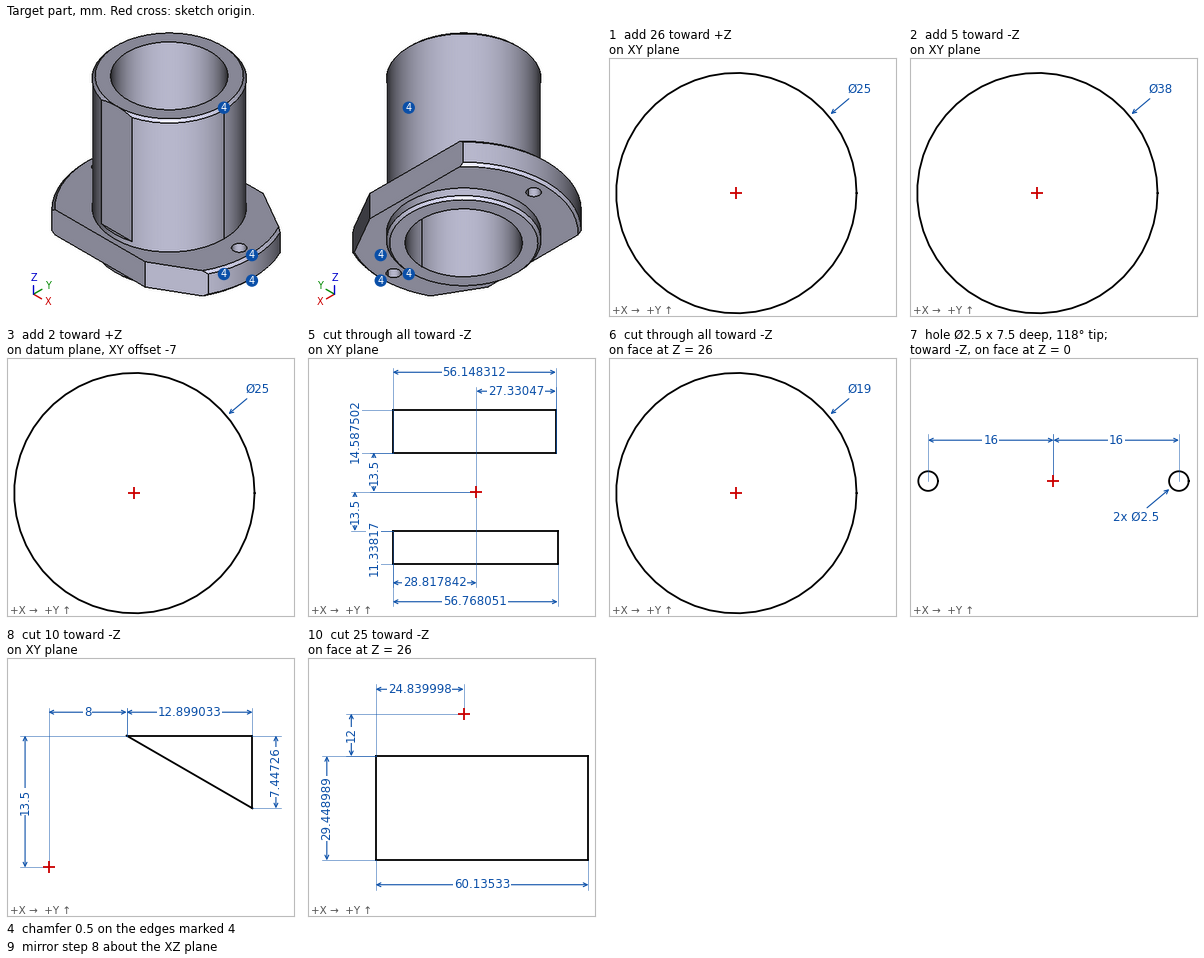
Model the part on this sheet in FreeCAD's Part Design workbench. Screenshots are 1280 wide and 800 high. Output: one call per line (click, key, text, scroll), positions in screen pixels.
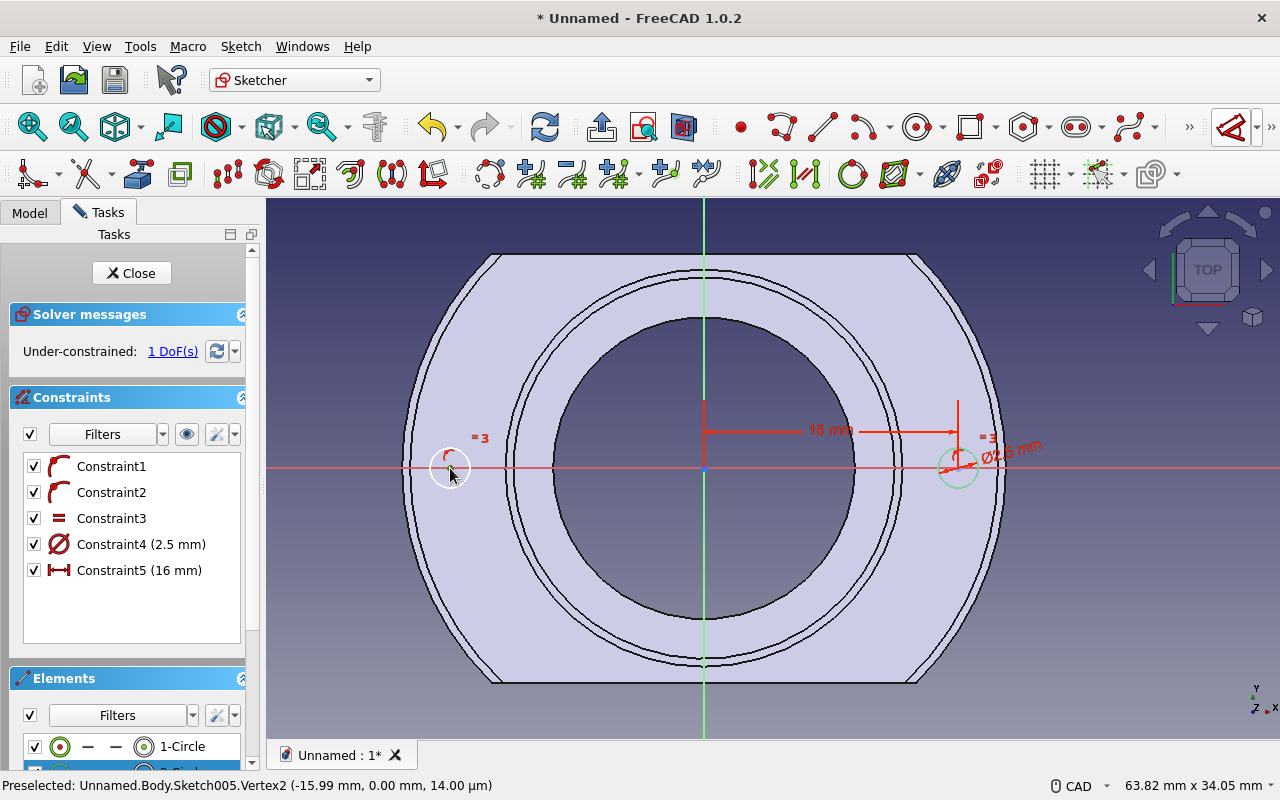
key(l)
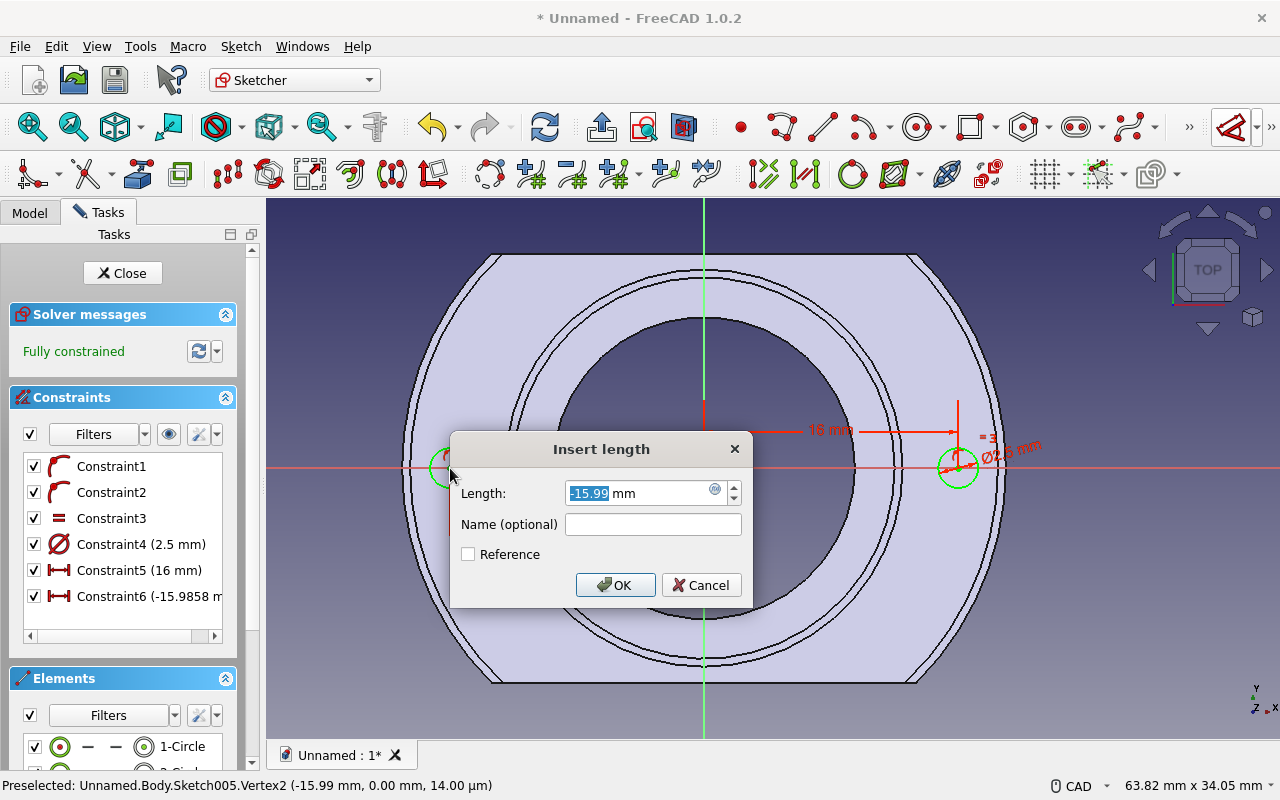
text(-16)
key(Return)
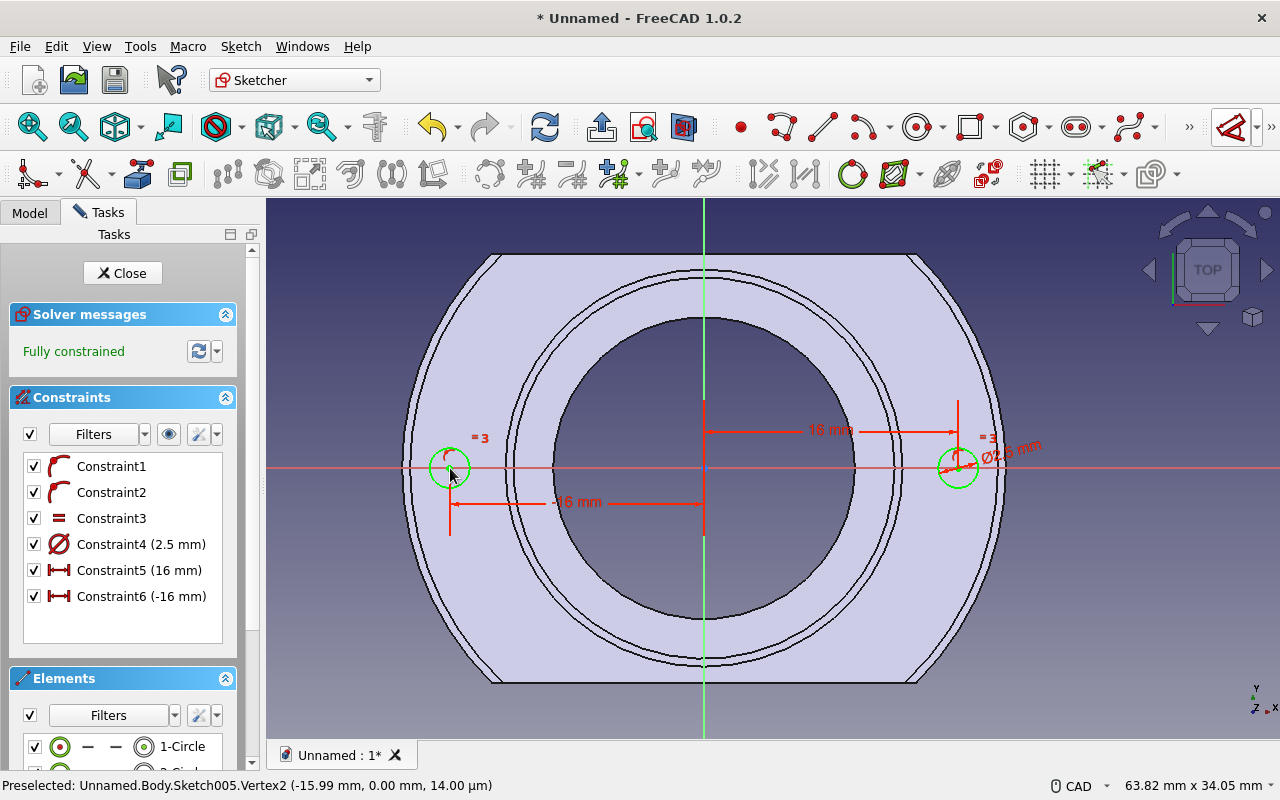
click(123, 273)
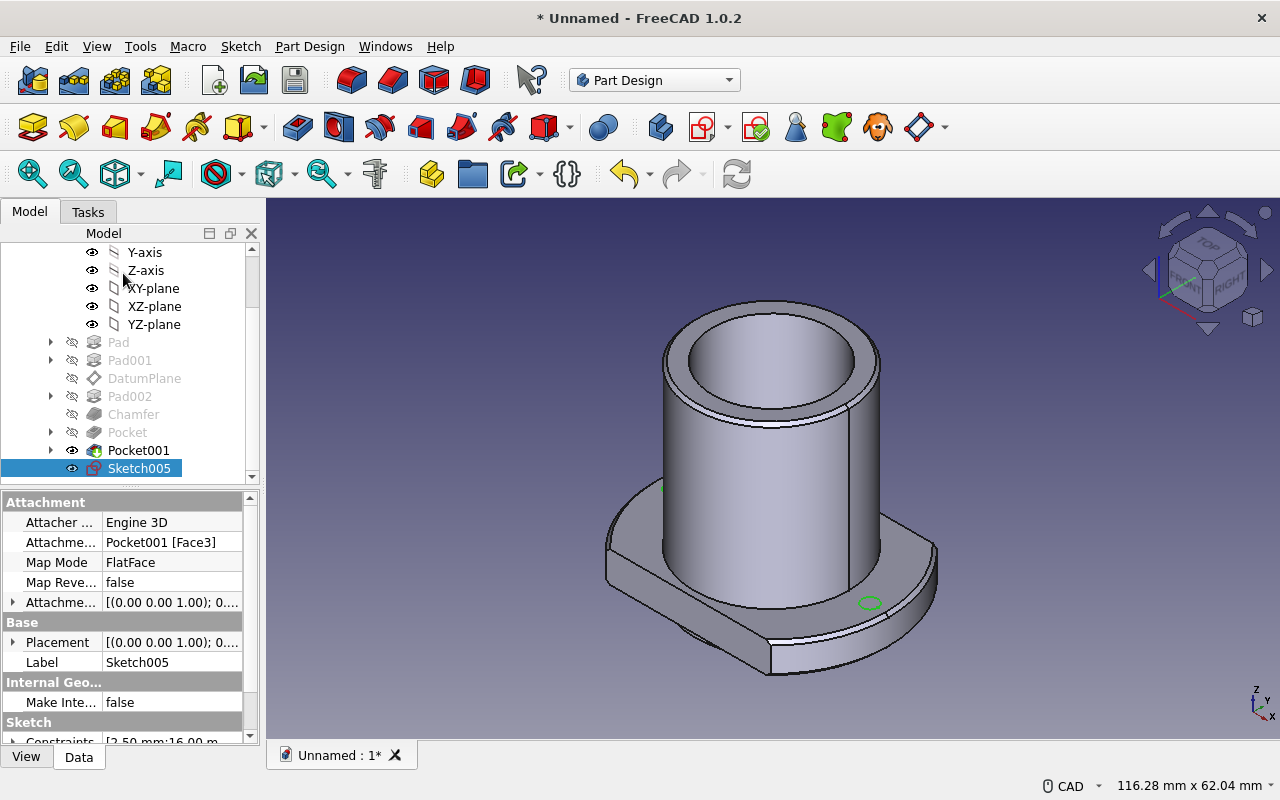
click(339, 128)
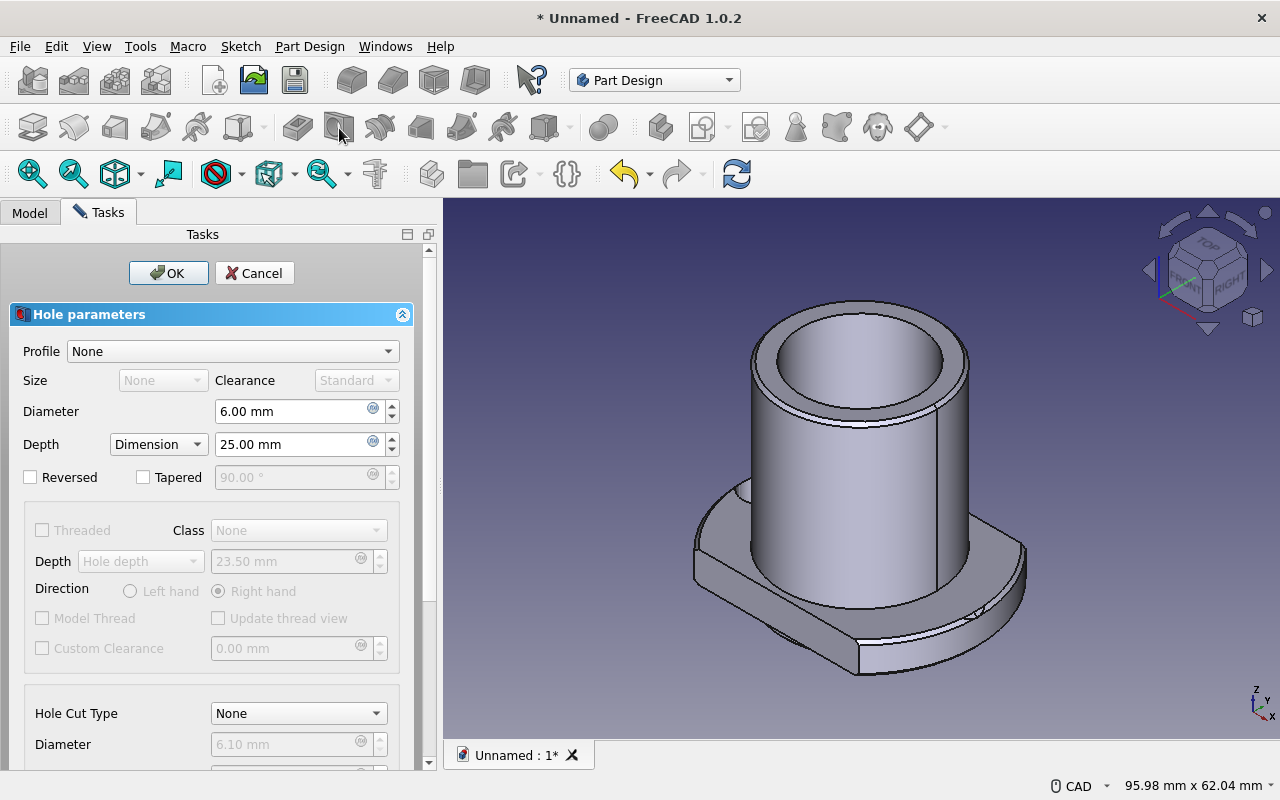
triple_click(300, 412)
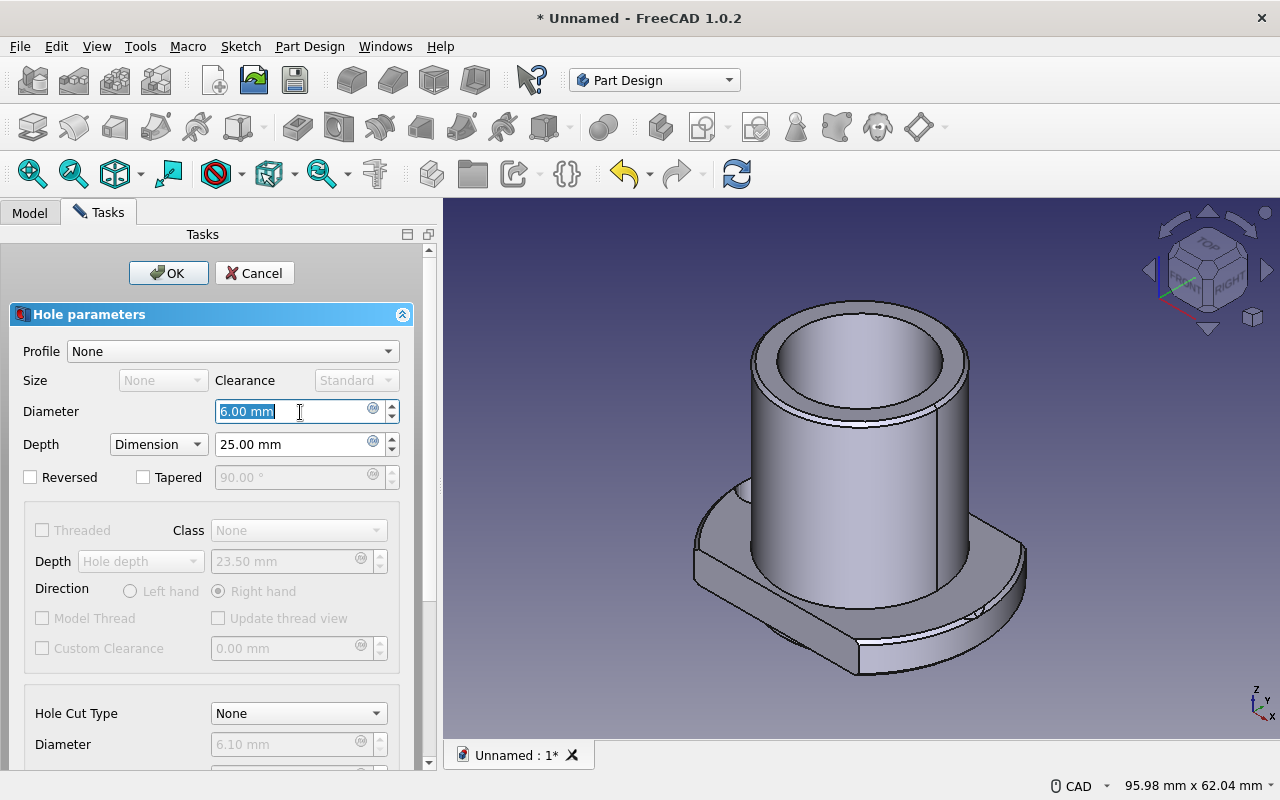
text(2.5)
key(Tab)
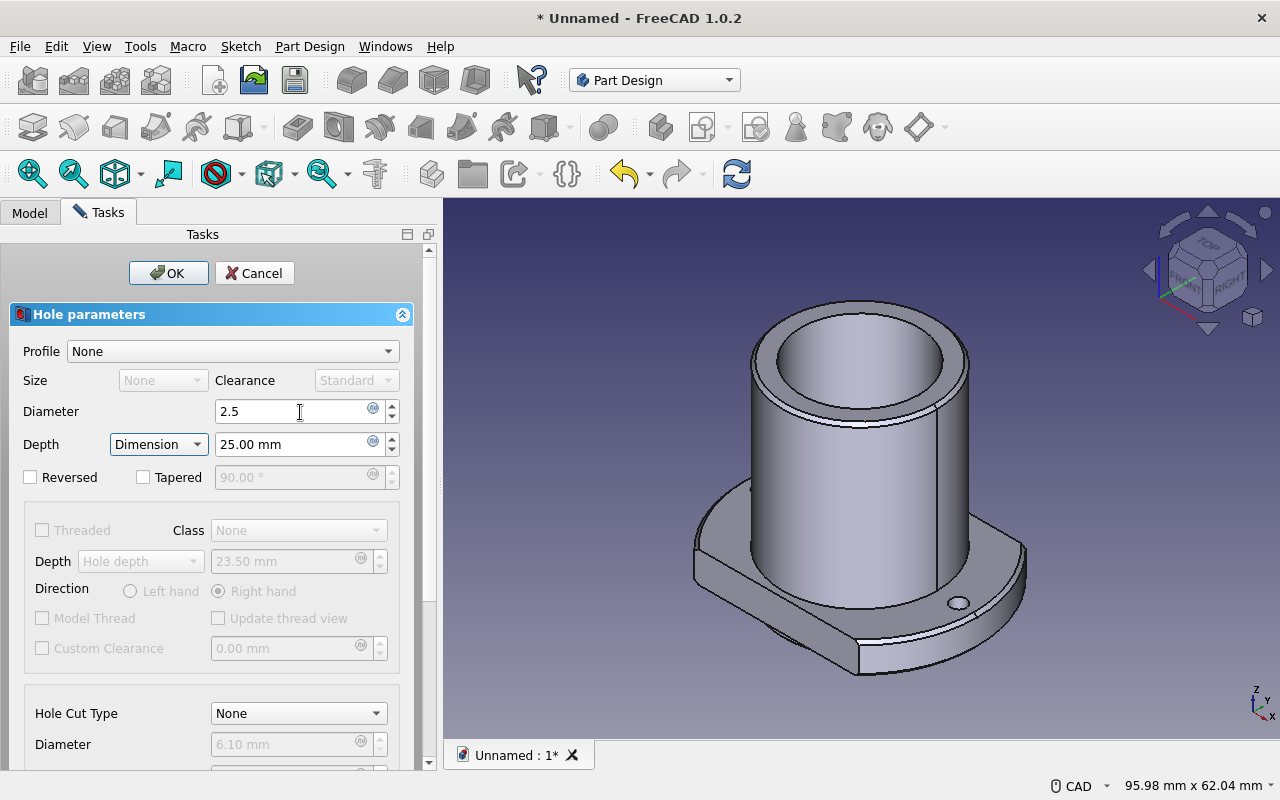
triple_click(300, 444)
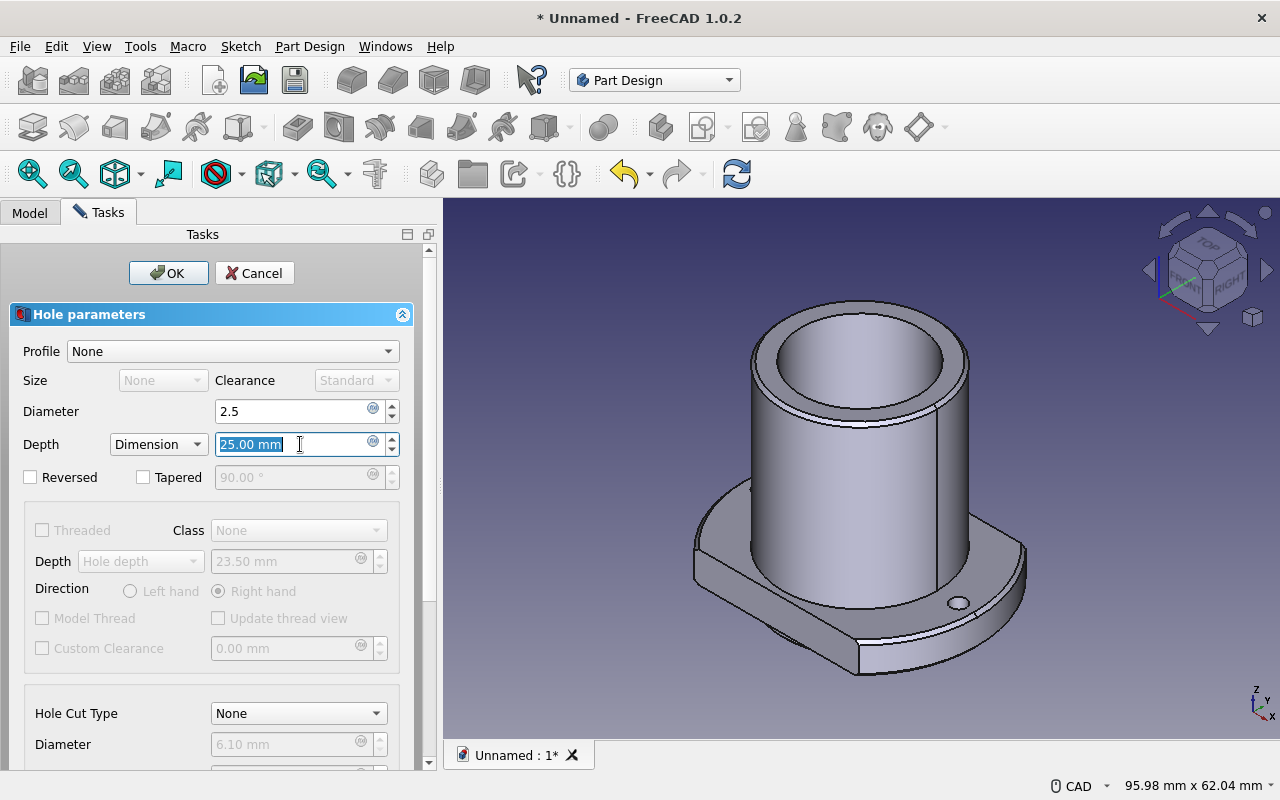
text(7.5)
key(Tab)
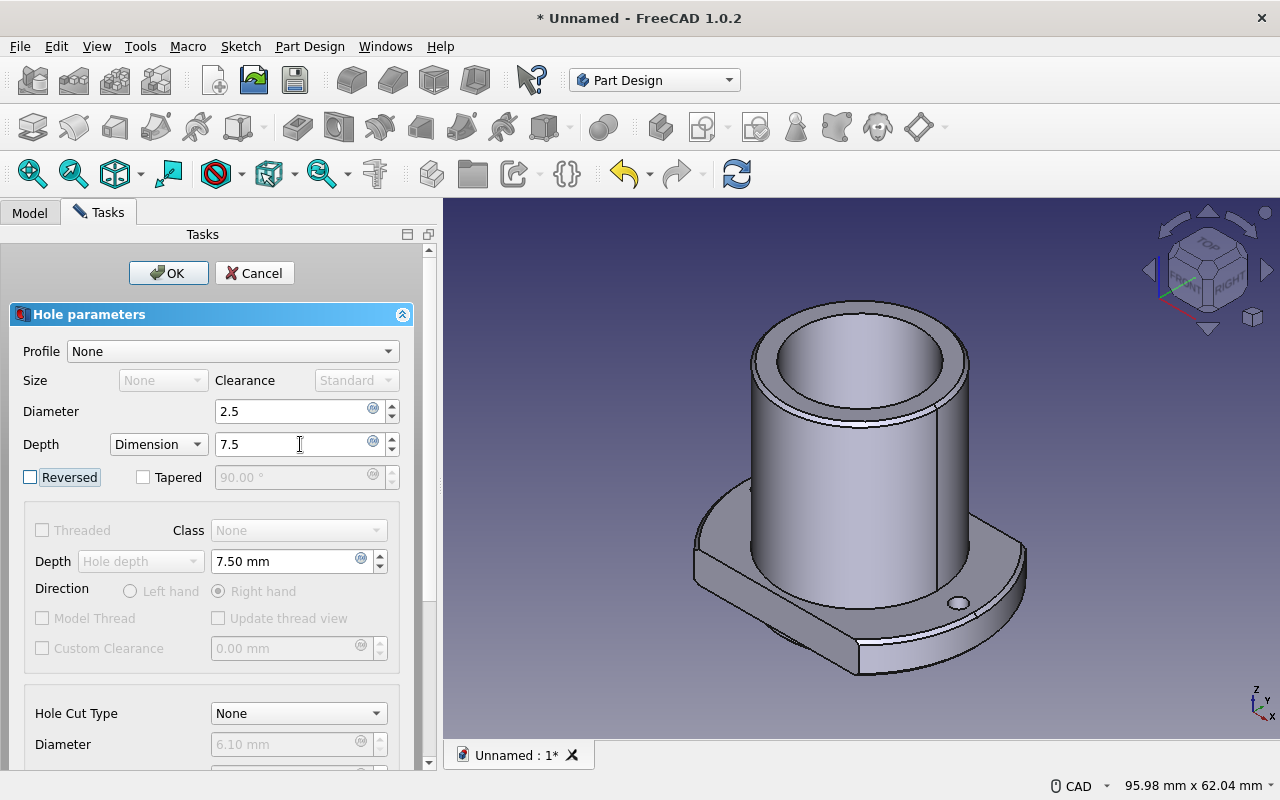
click(169, 273)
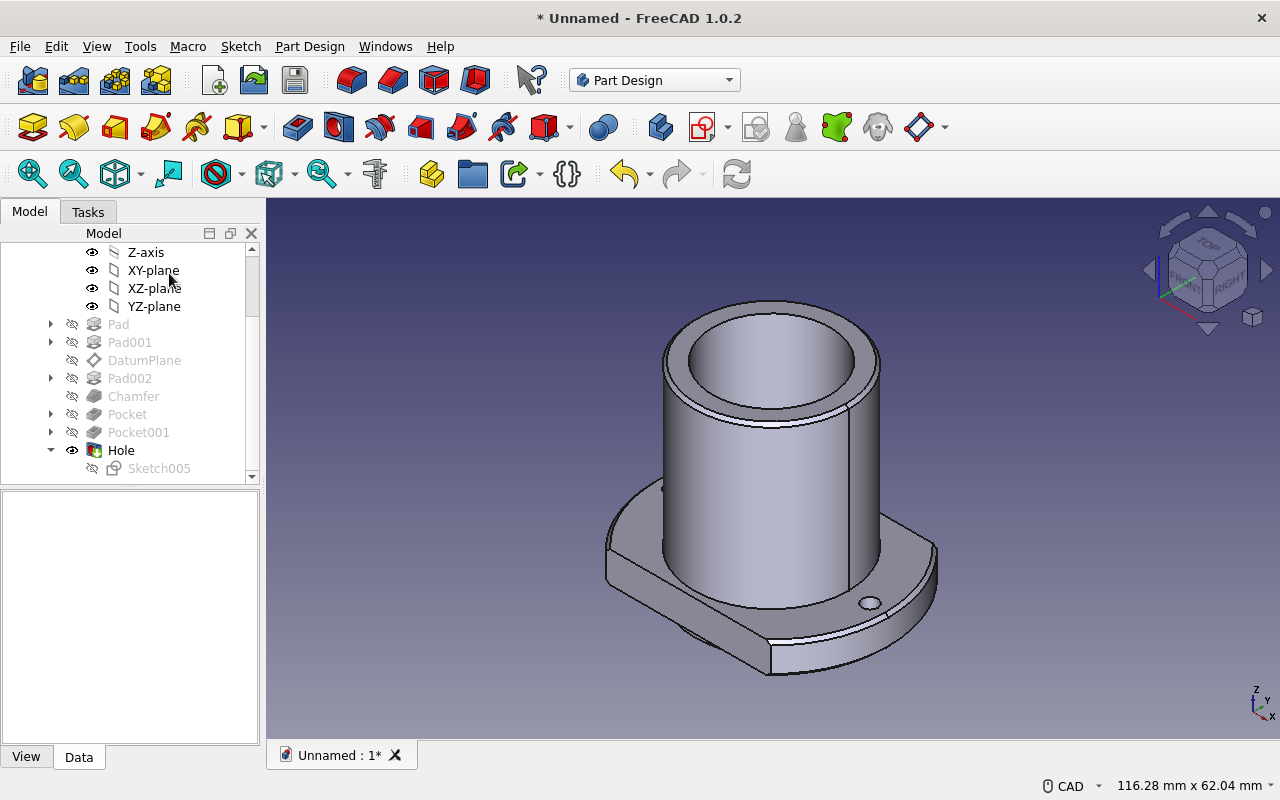
click(702, 128)